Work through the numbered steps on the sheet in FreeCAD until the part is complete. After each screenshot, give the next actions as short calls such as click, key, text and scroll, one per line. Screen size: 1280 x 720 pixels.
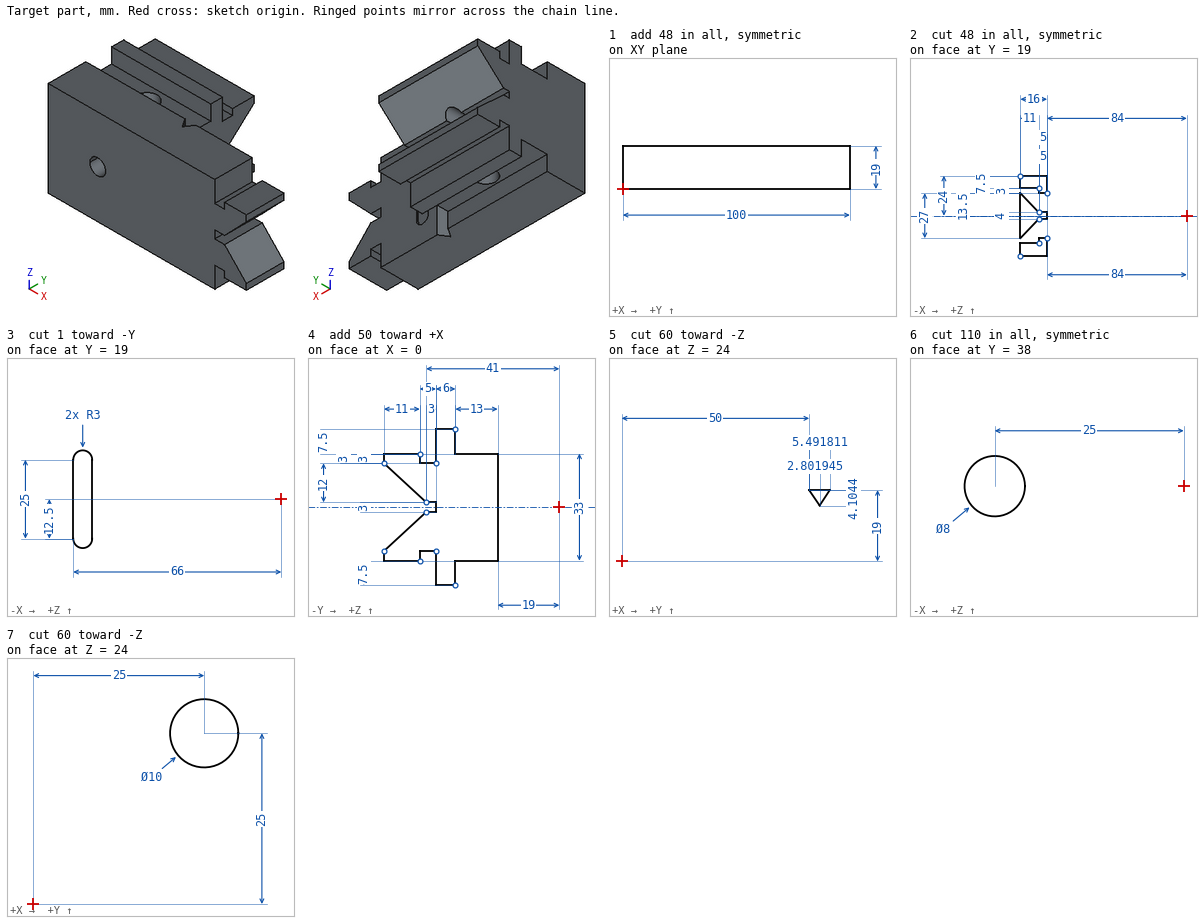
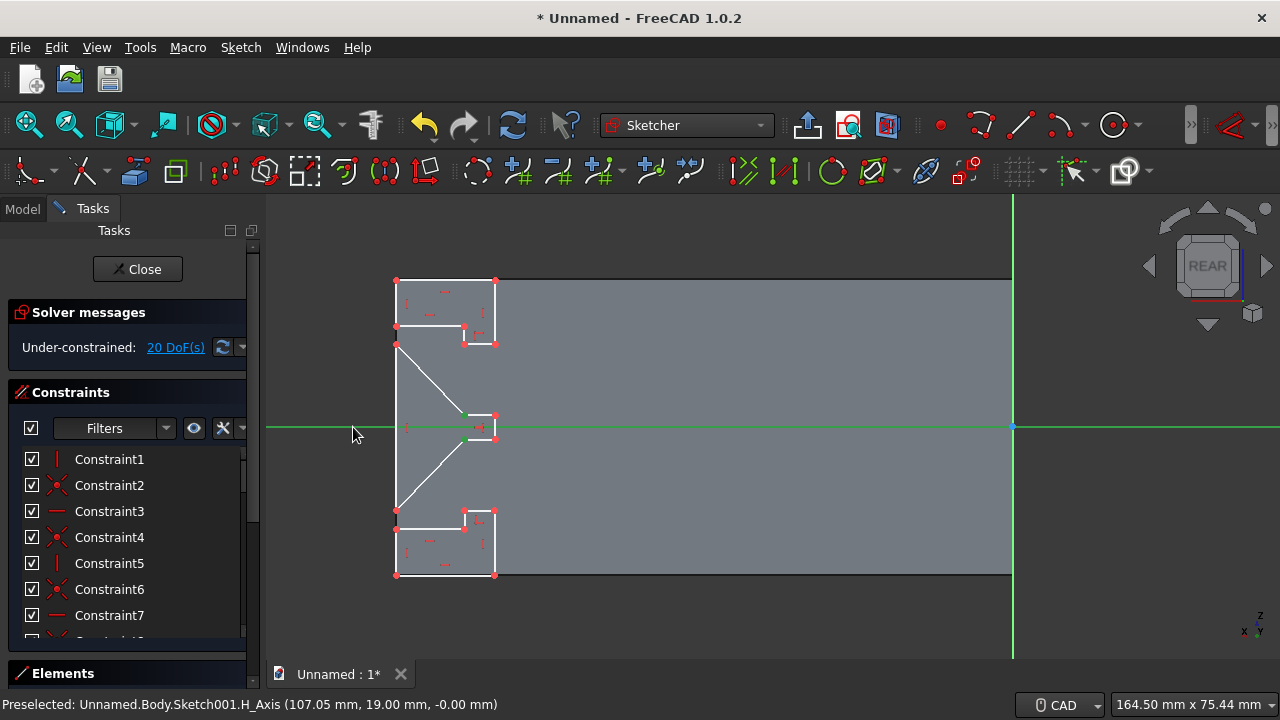
key(s)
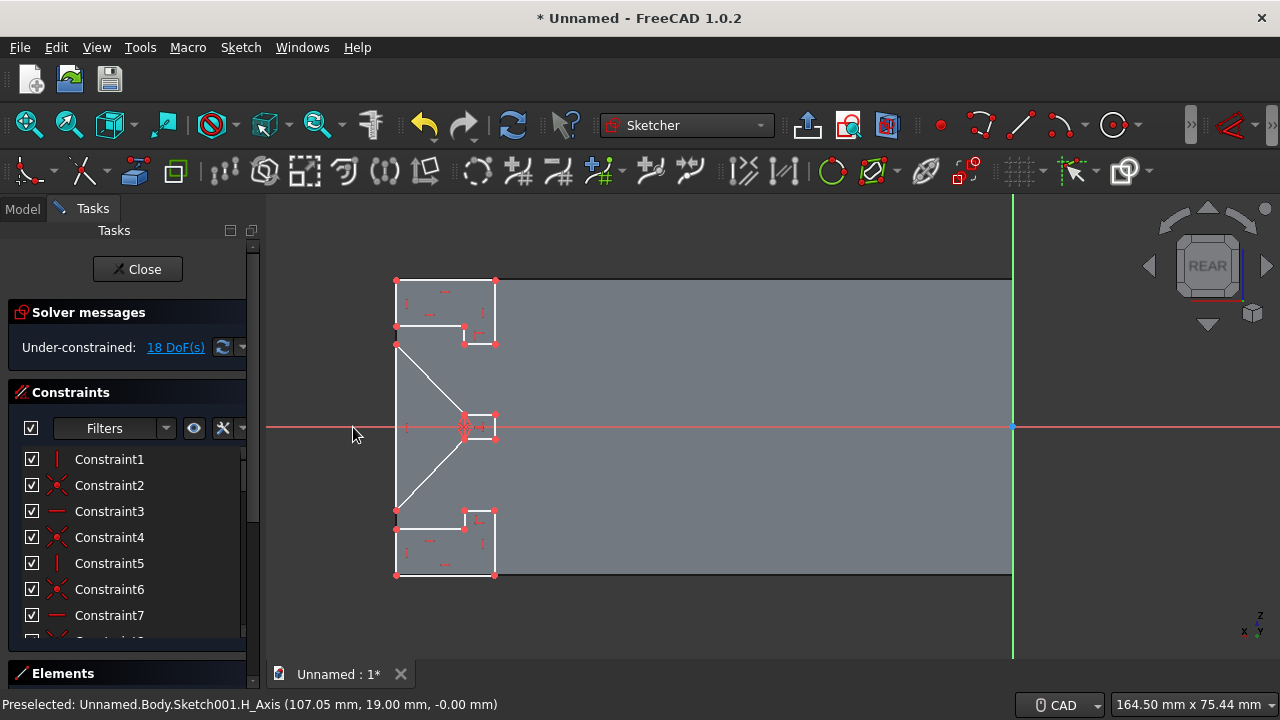
click(495, 344)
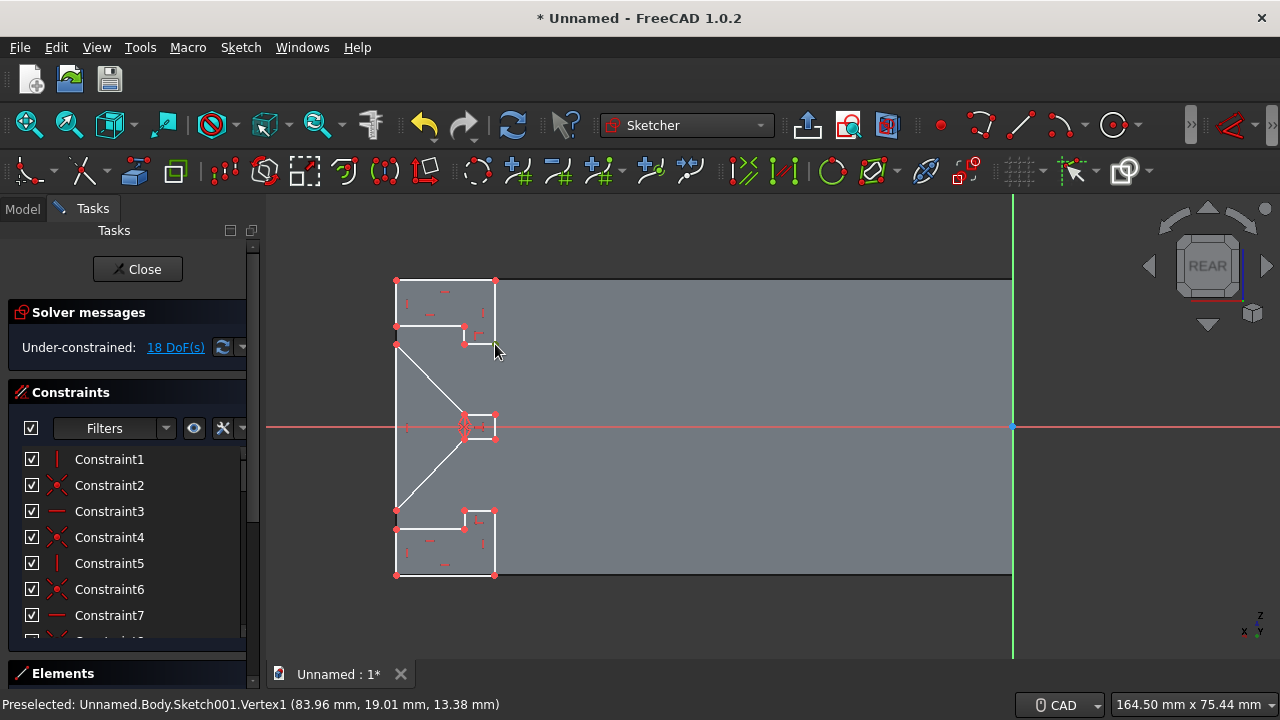
click(495, 511)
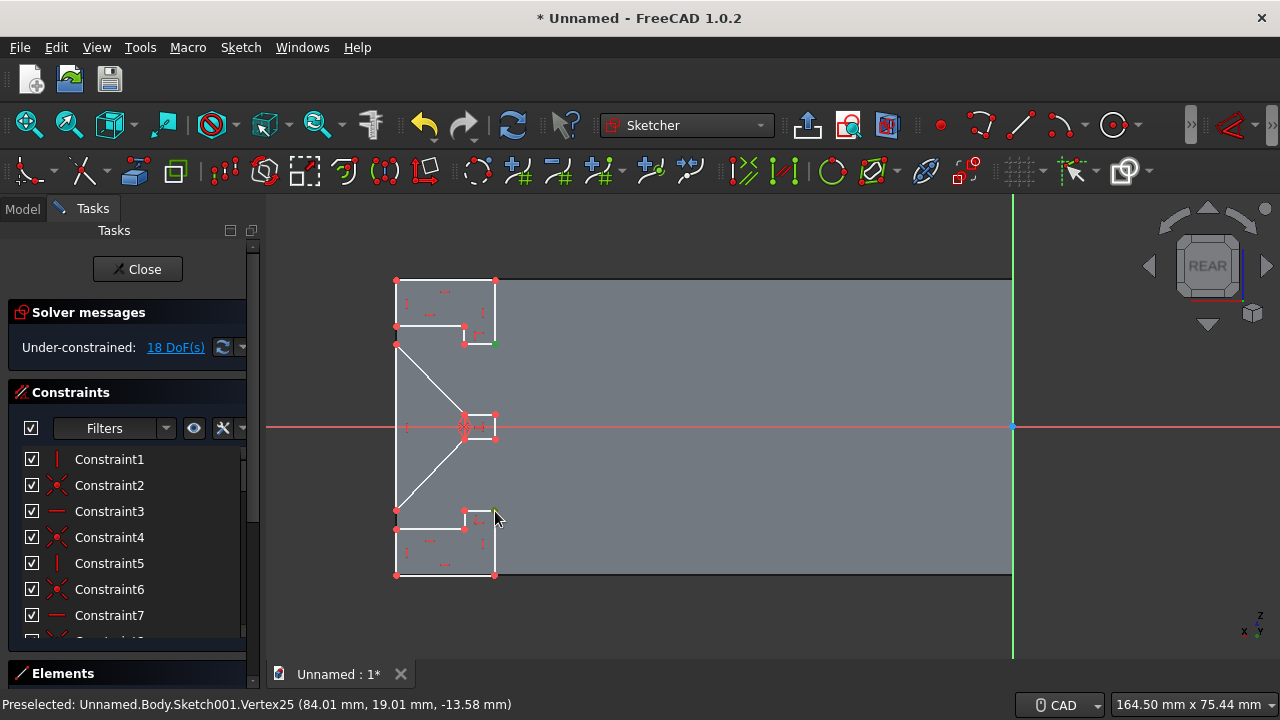
click(353, 427)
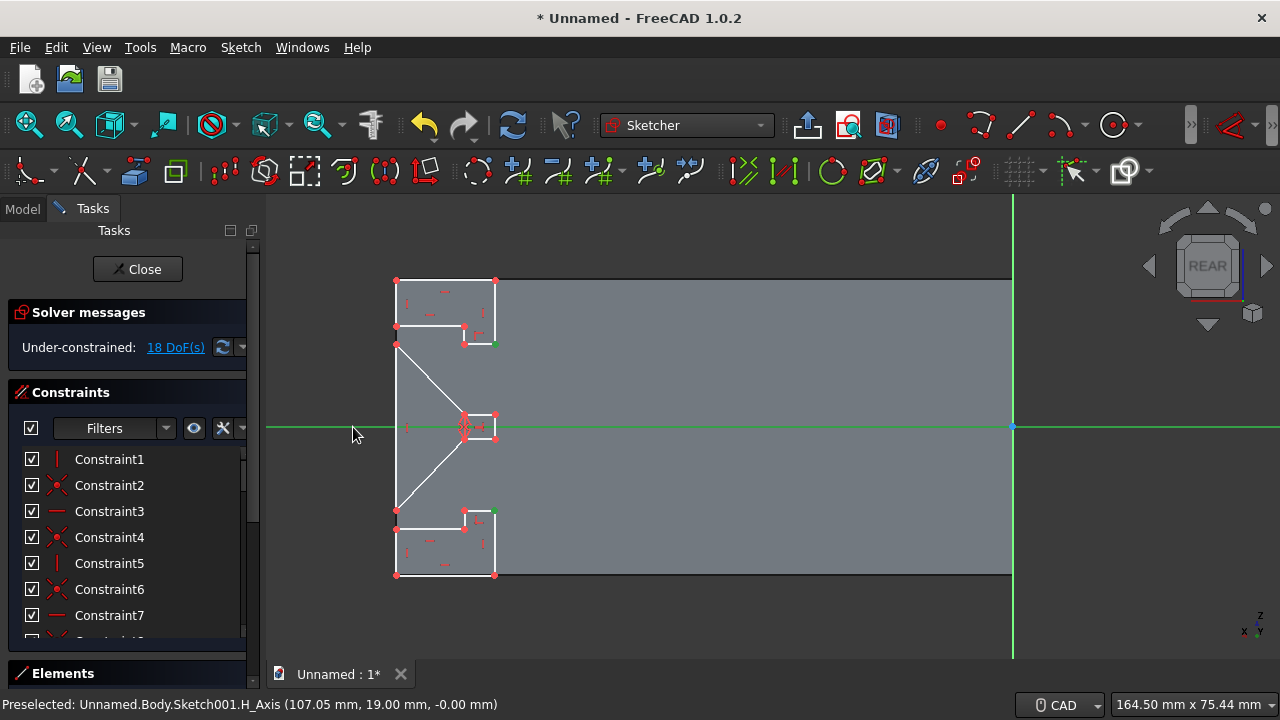
key(s)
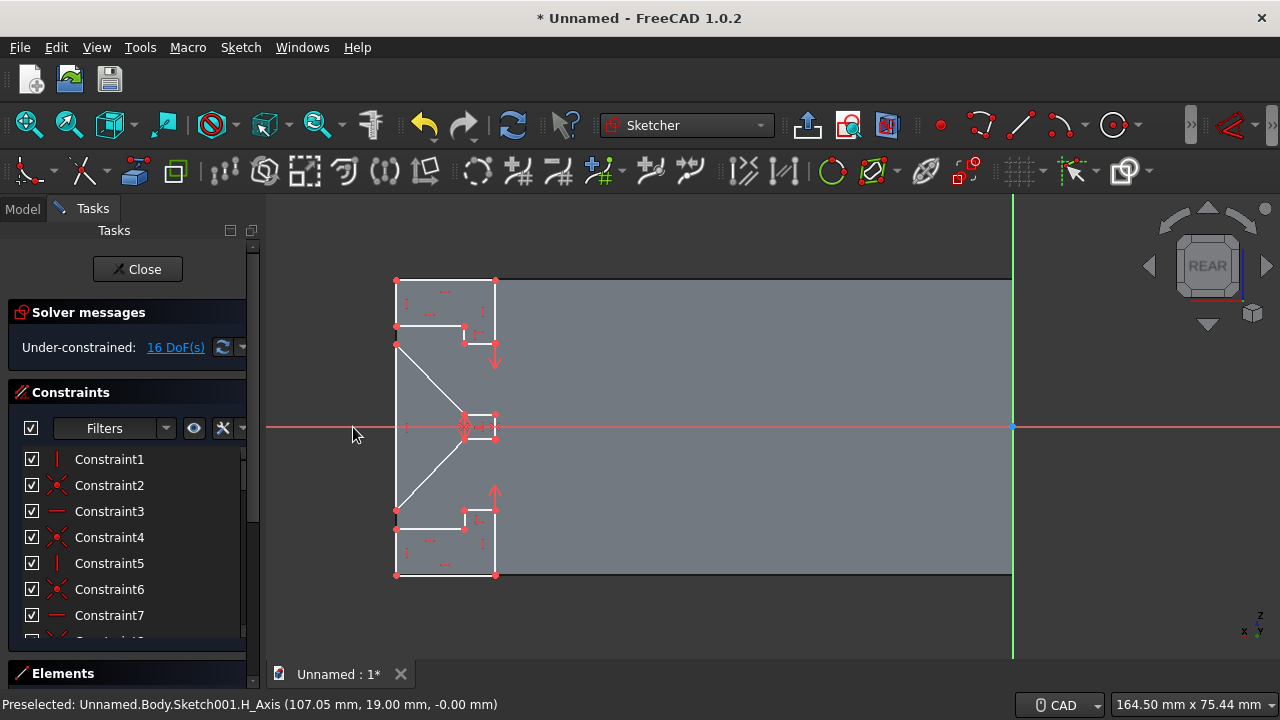
click(464, 326)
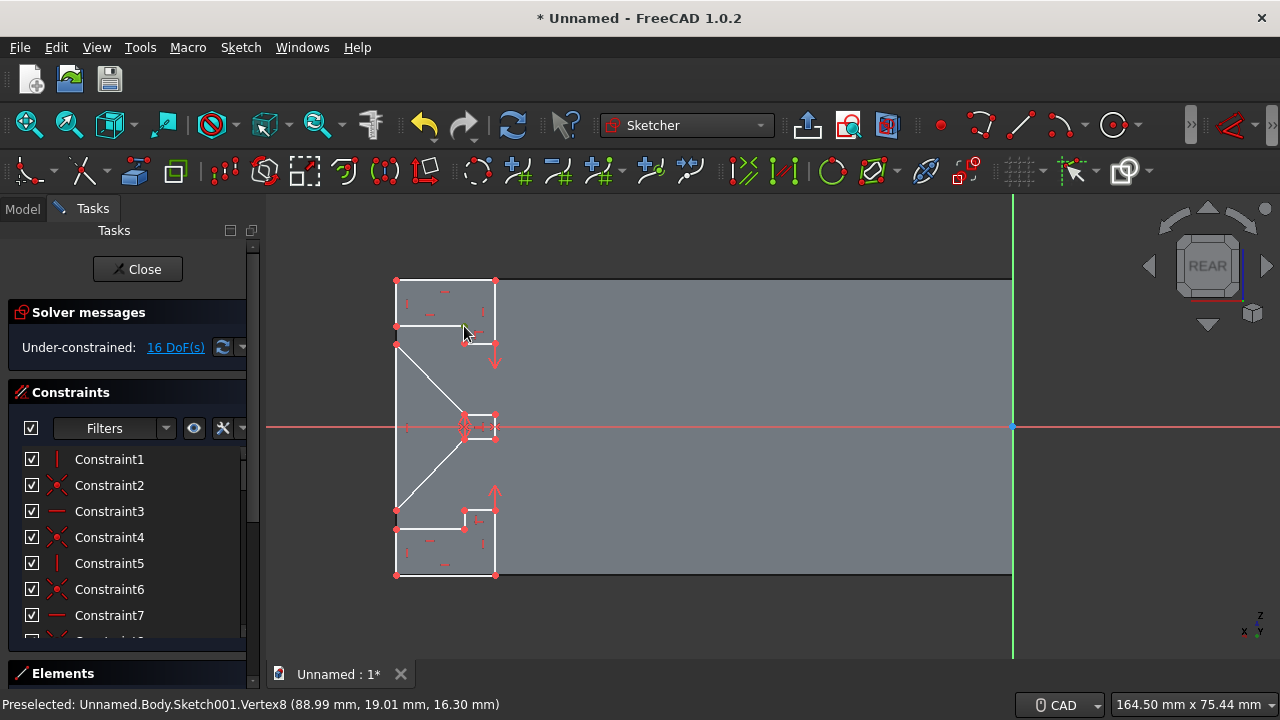
click(465, 529)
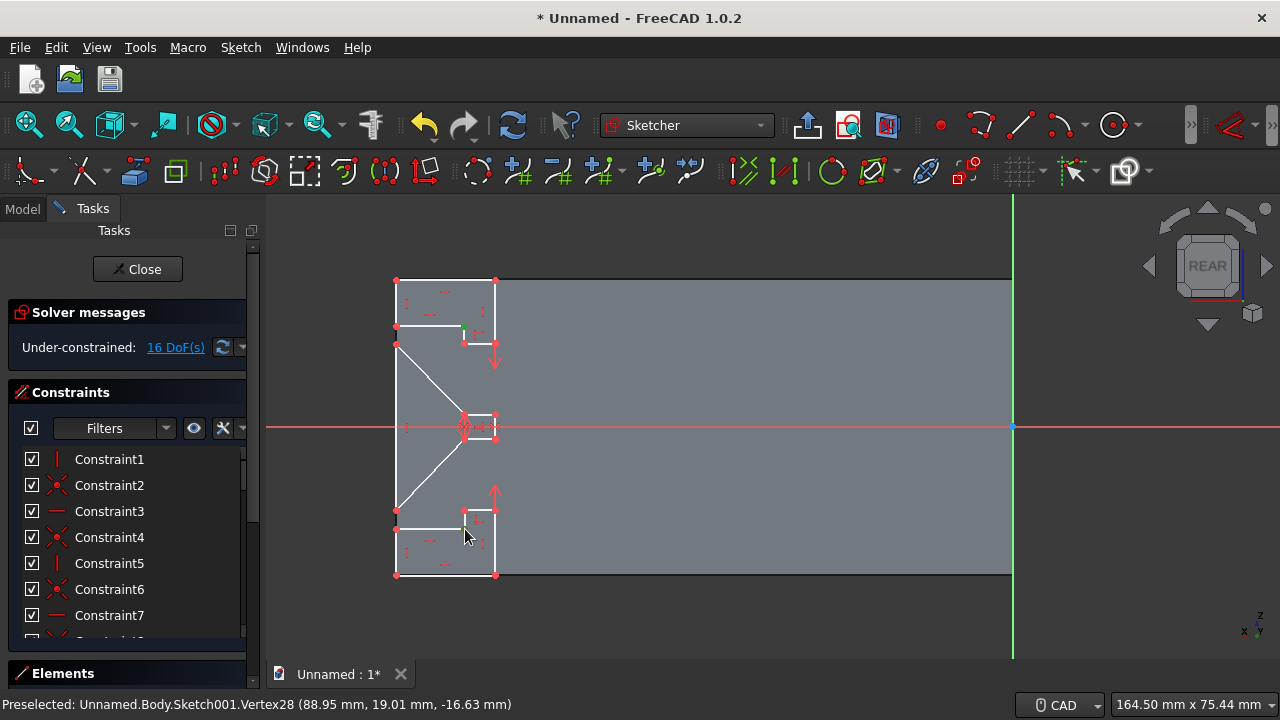
click(353, 427)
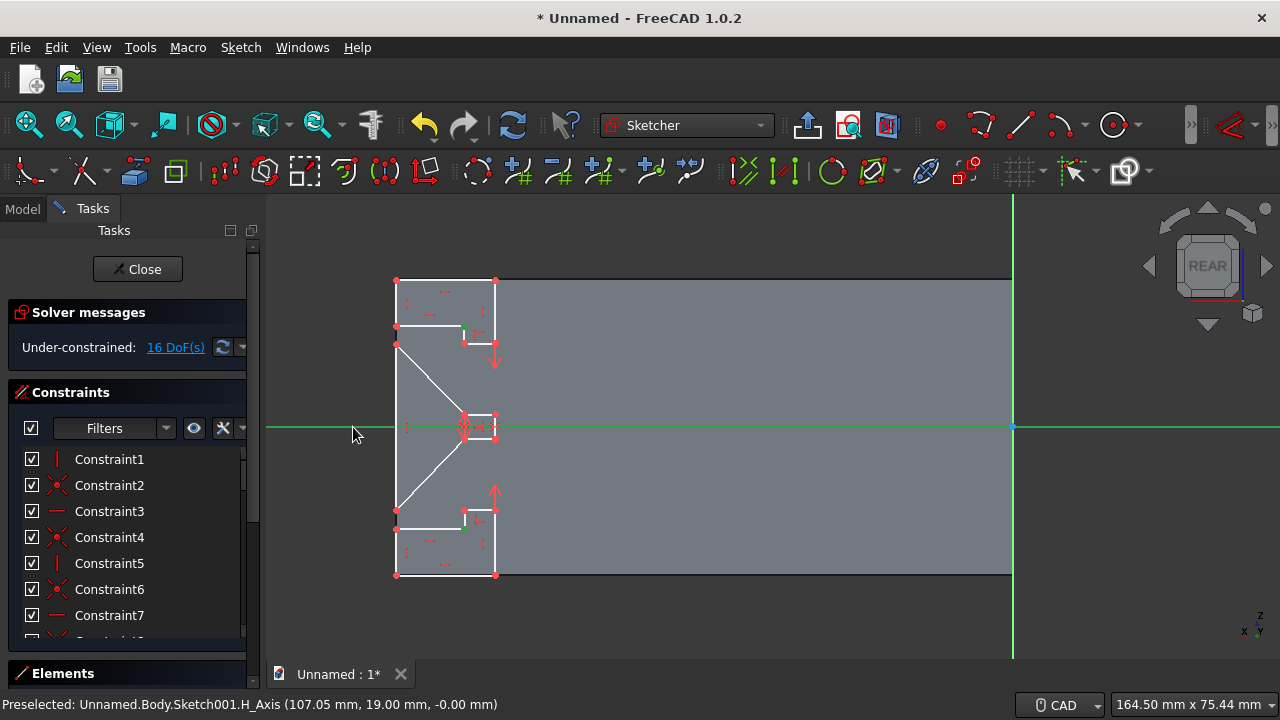
key(s)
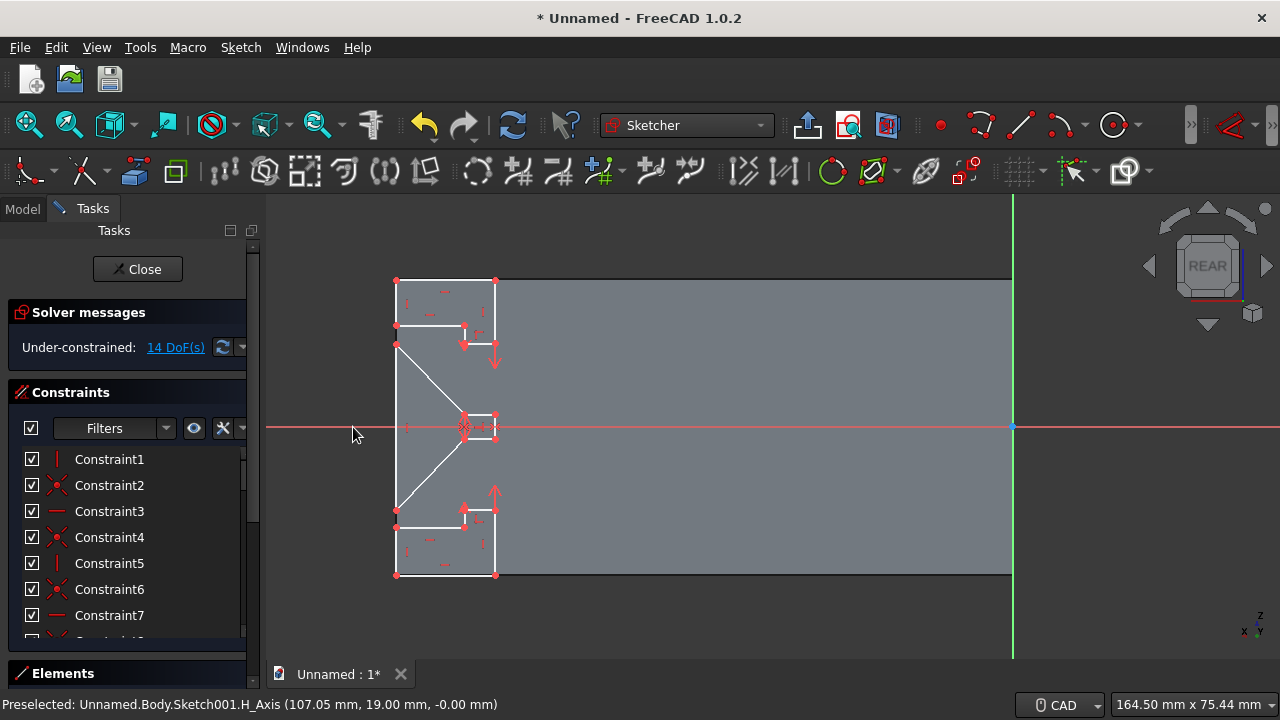
click(396, 280)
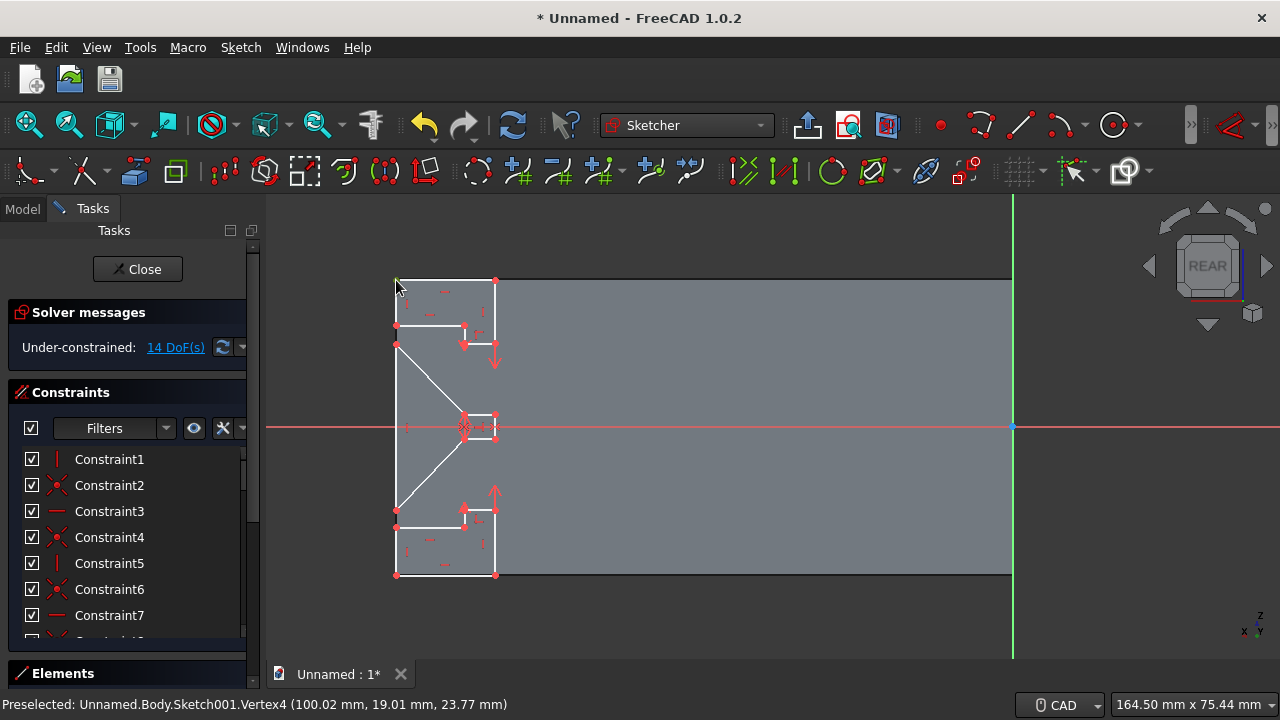
click(396, 576)